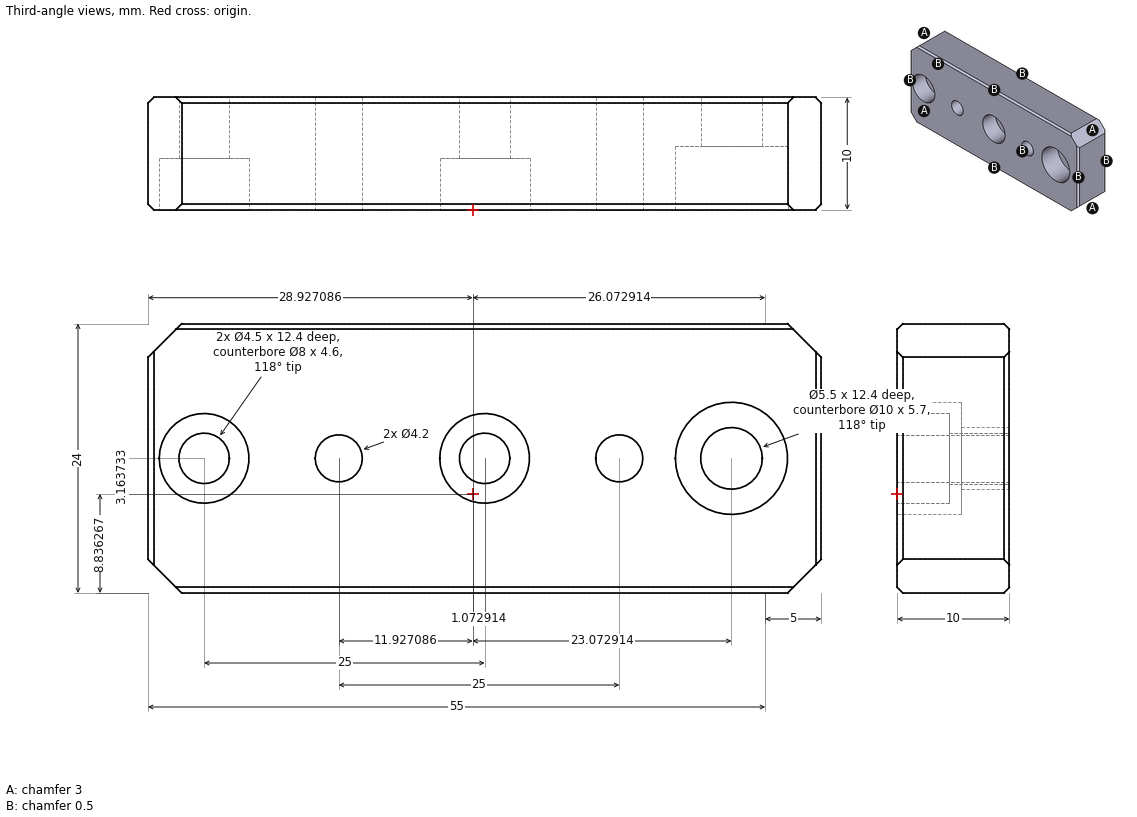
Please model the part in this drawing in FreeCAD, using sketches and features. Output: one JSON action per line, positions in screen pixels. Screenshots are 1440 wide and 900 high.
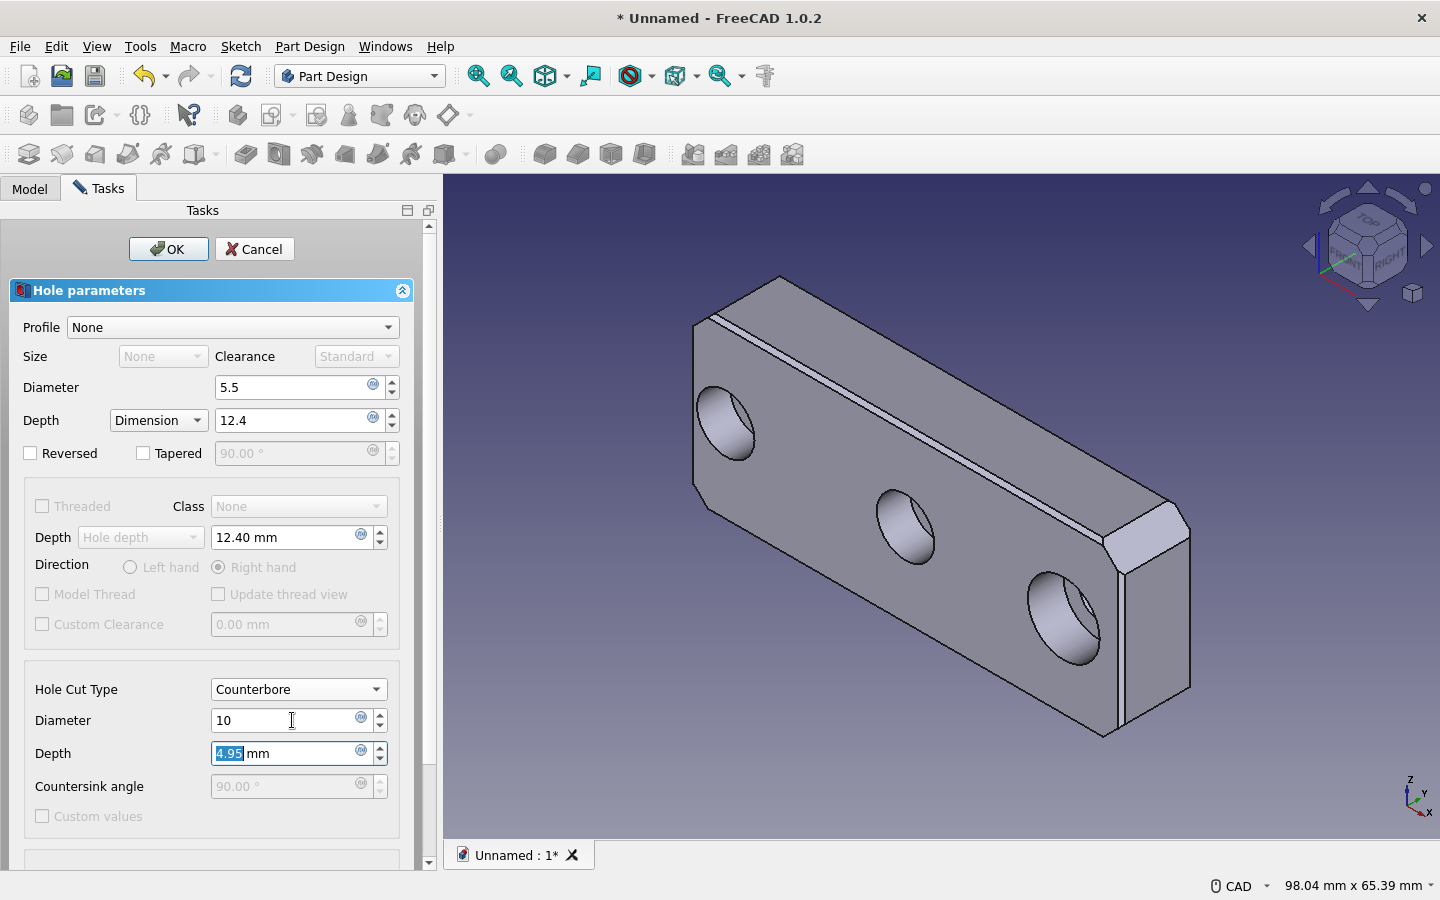
{"action": "type", "text": "5.7"}
{"action": "key", "text": "Tab"}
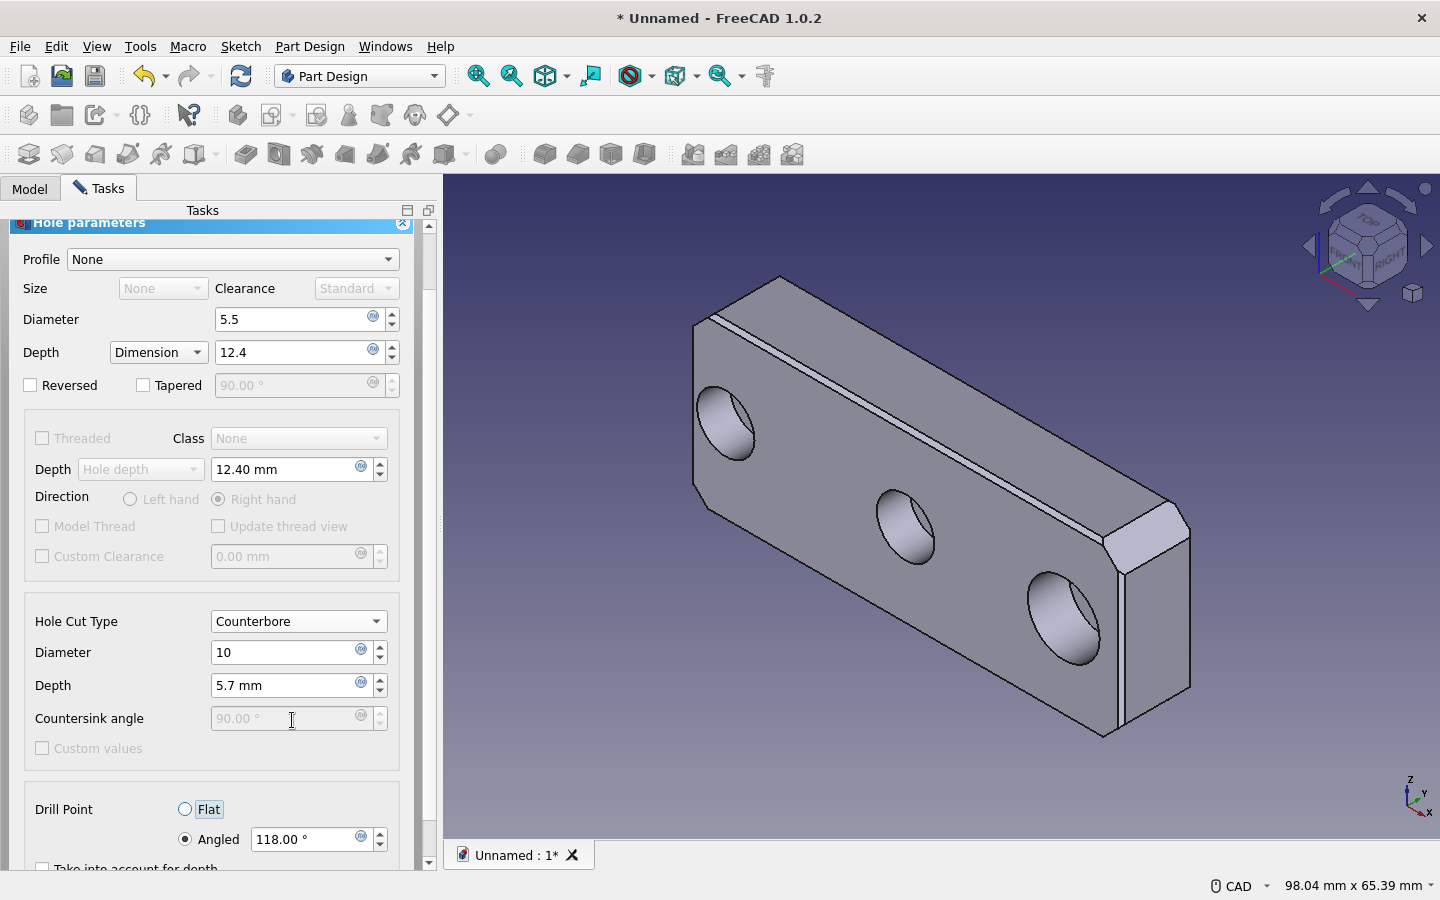
{"action": "scroll", "coordinate": [429, 545], "scroll_direction": "up", "scroll_amount": 2}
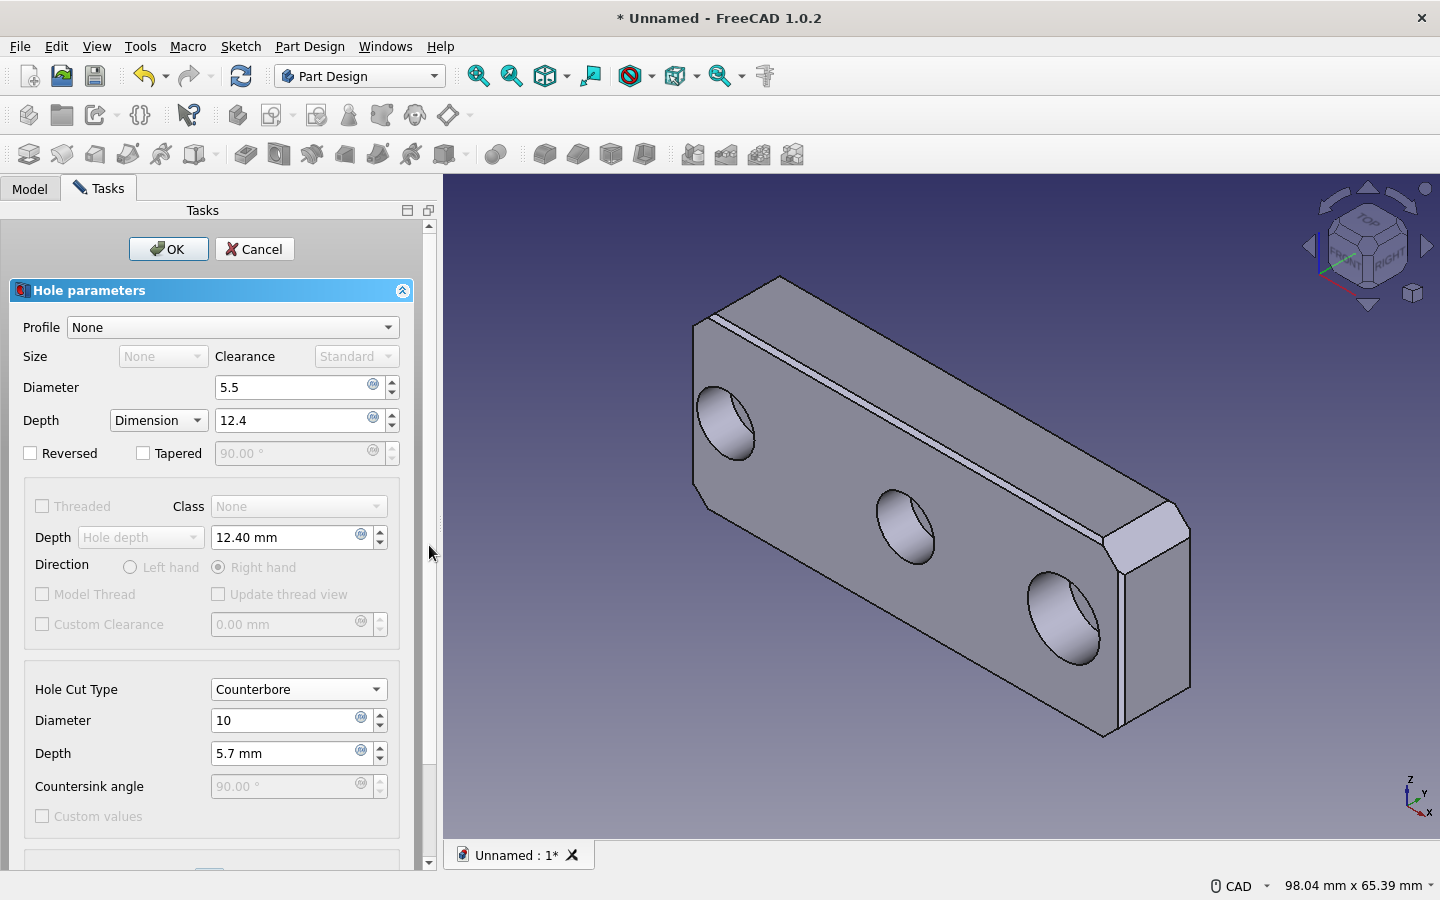
{"action": "left_click", "coordinate": [169, 249]}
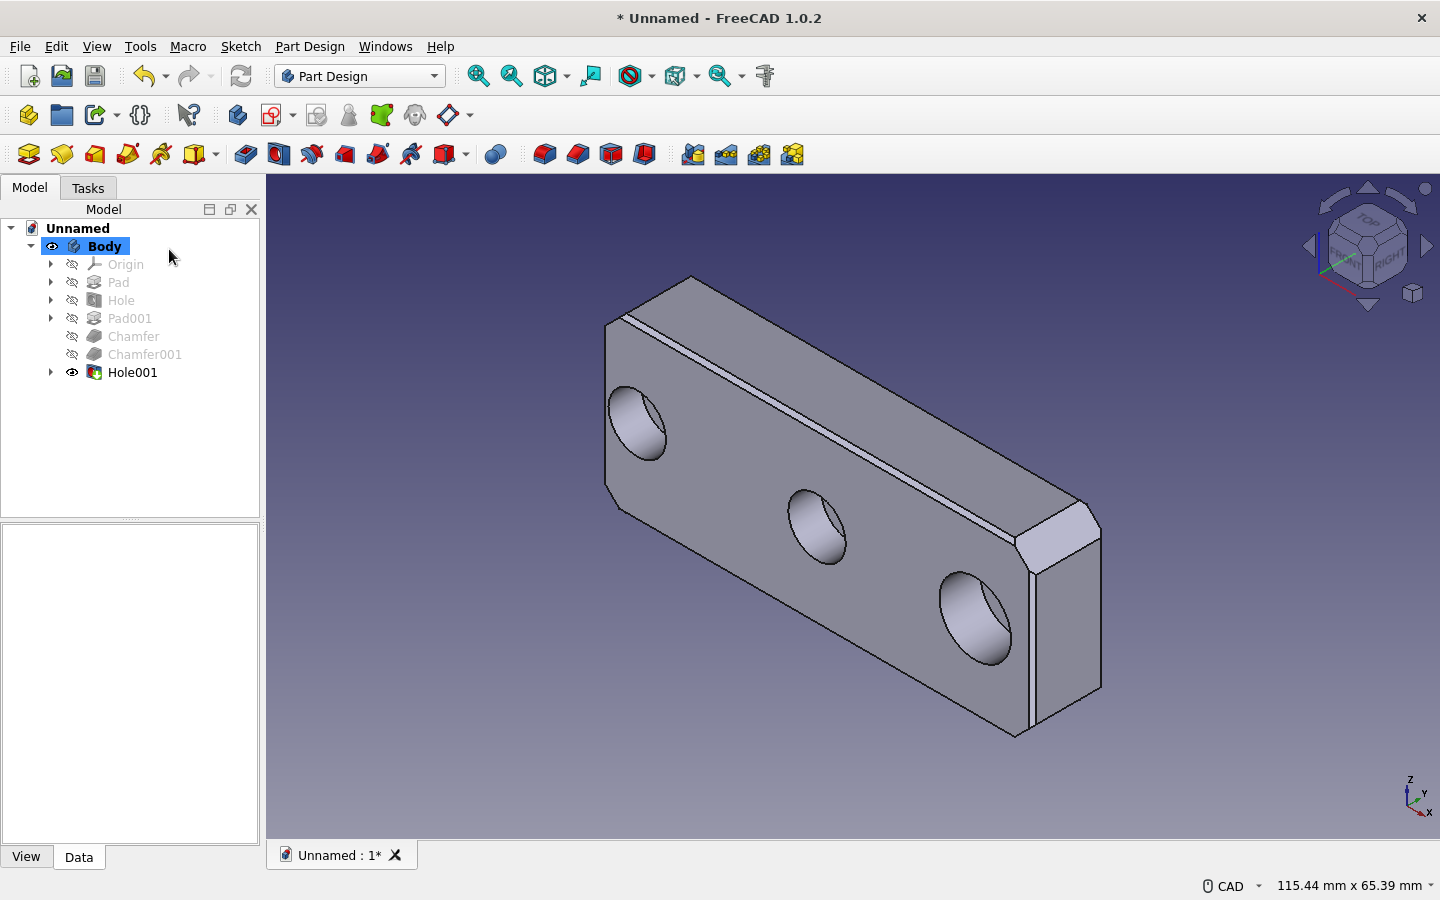
{"action": "key", "text": "4"}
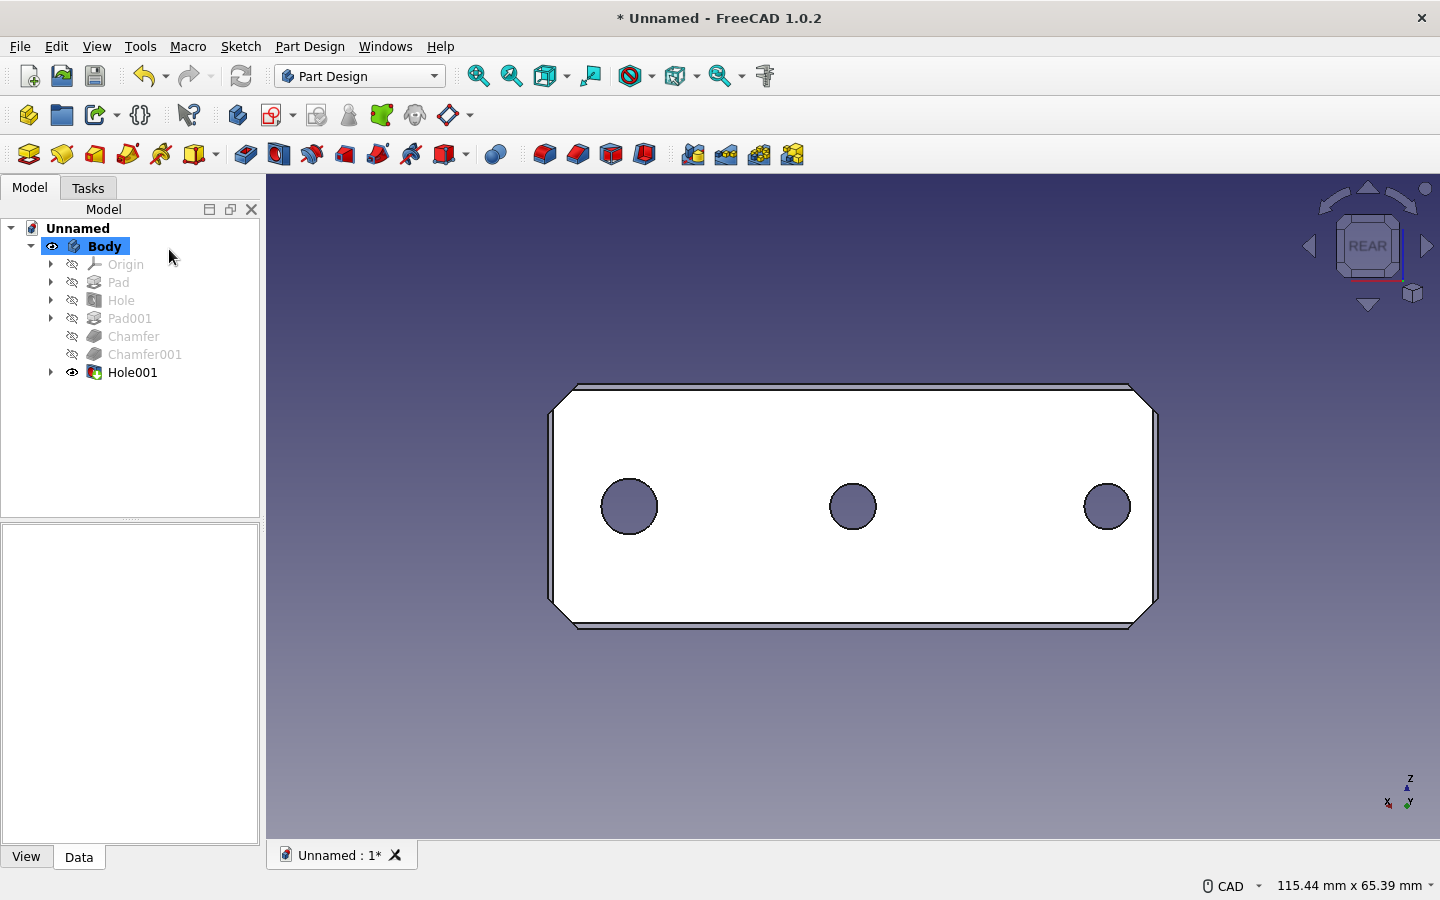
{"action": "left_click", "coordinate": [939, 472]}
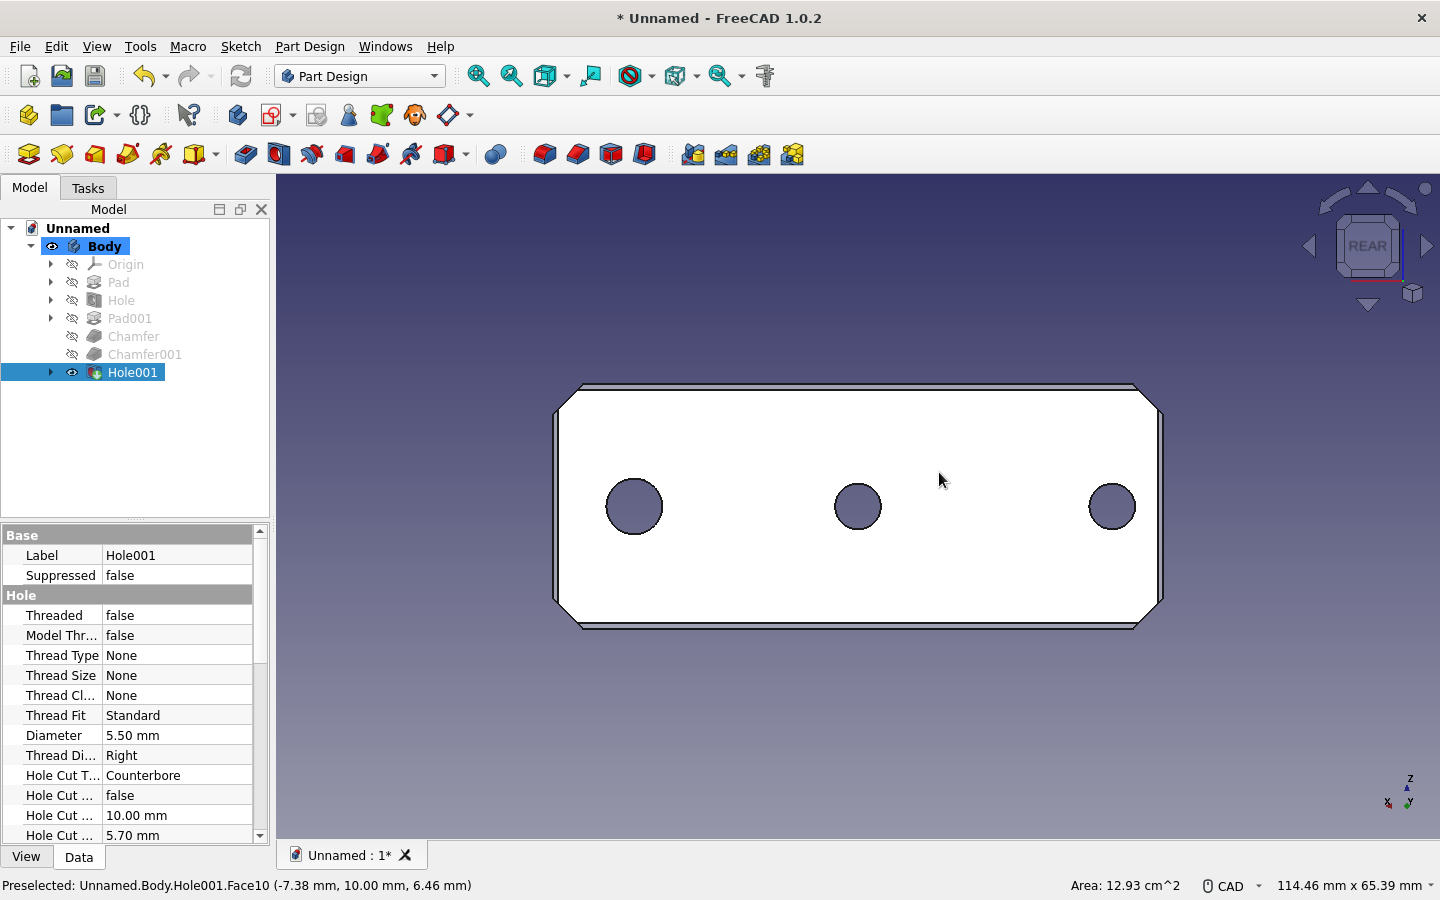
{"action": "left_click", "coordinate": [270, 116]}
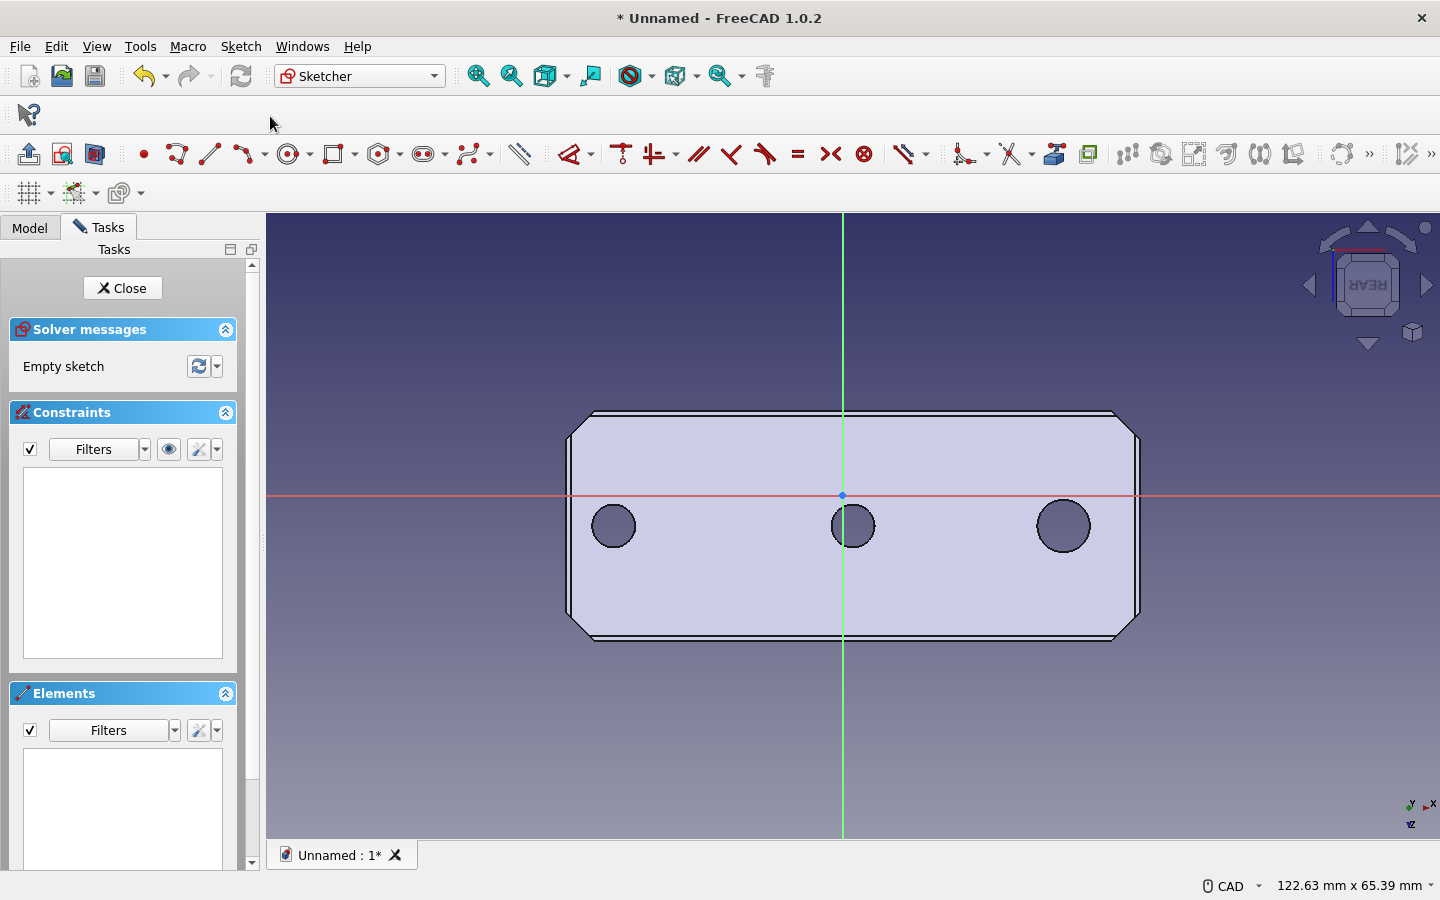
{"action": "scroll", "coordinate": [885, 518], "scroll_direction": "up", "scroll_amount": 5}